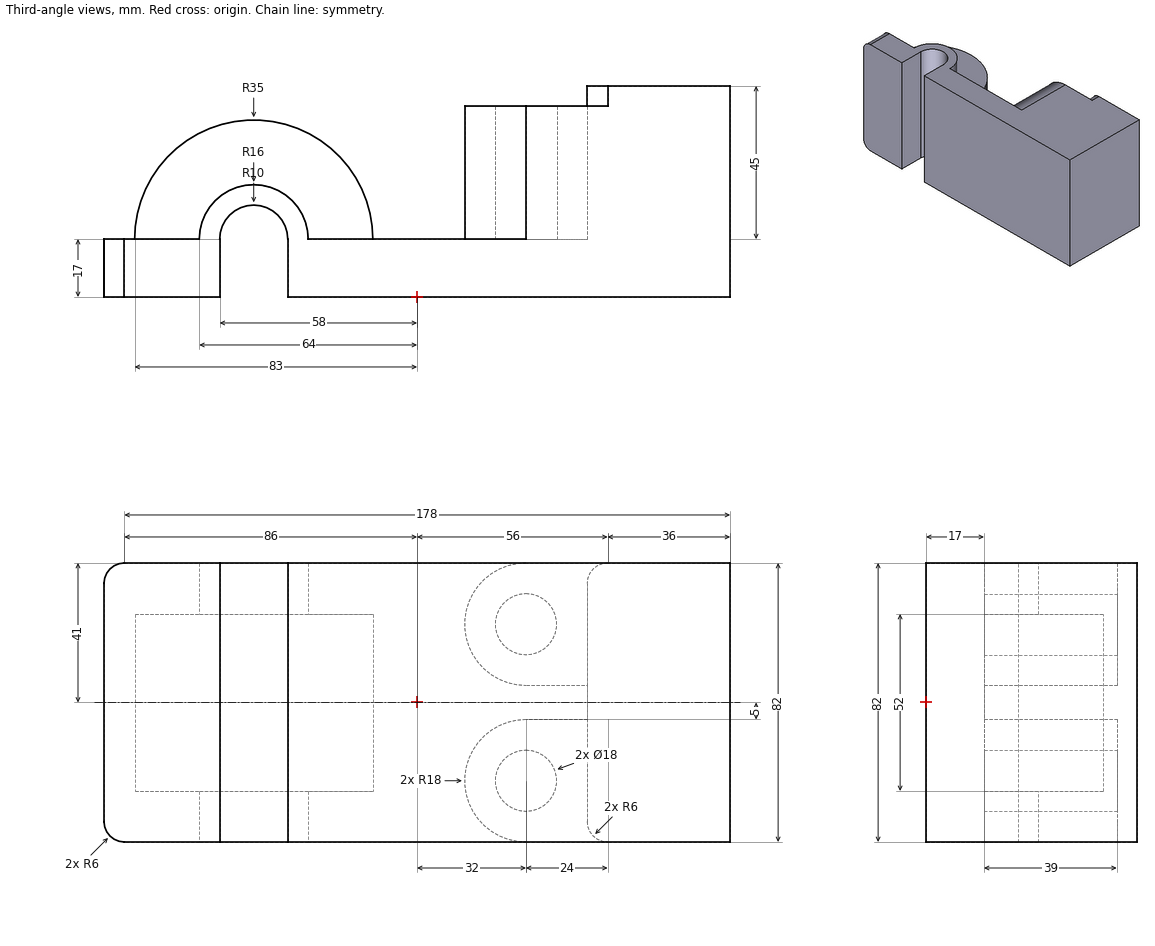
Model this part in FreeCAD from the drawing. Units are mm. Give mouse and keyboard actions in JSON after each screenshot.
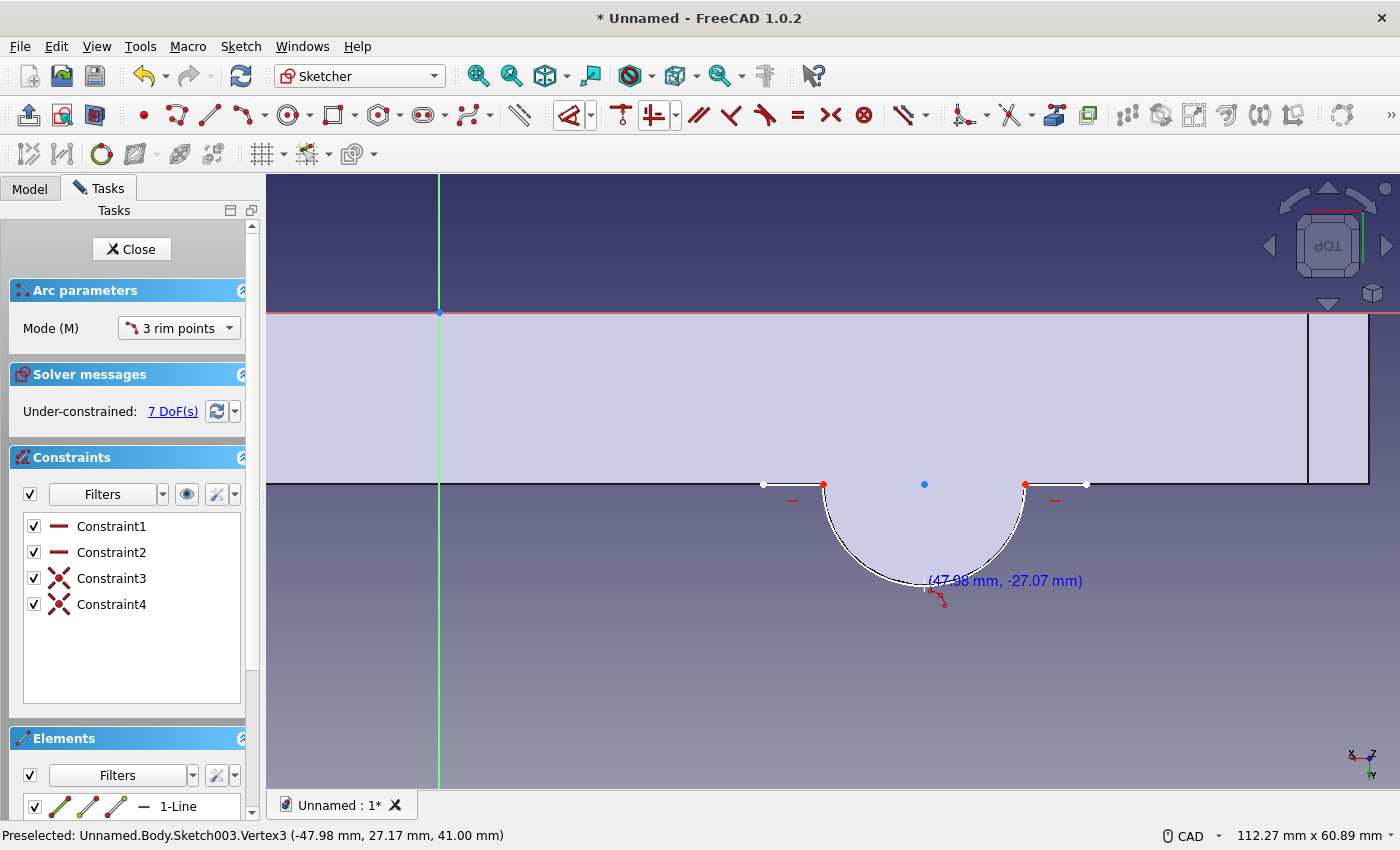
{"action": "left_click", "coordinate": [763, 485]}
{"action": "left_click", "coordinate": [1086, 485]}
{"action": "left_click", "coordinate": [924, 646]}
{"action": "key", "text": "Escape"}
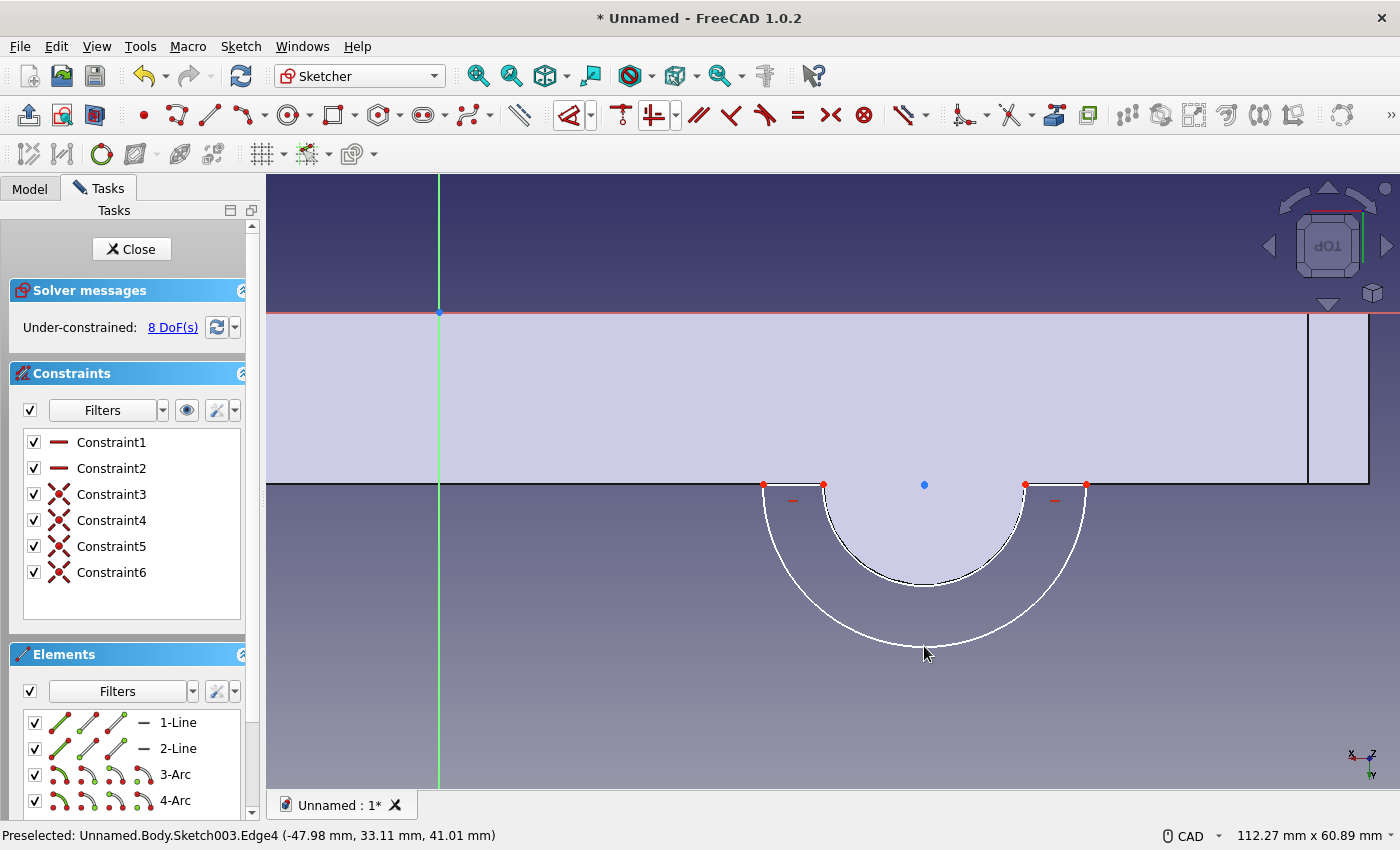
{"action": "left_click", "coordinate": [865, 567]}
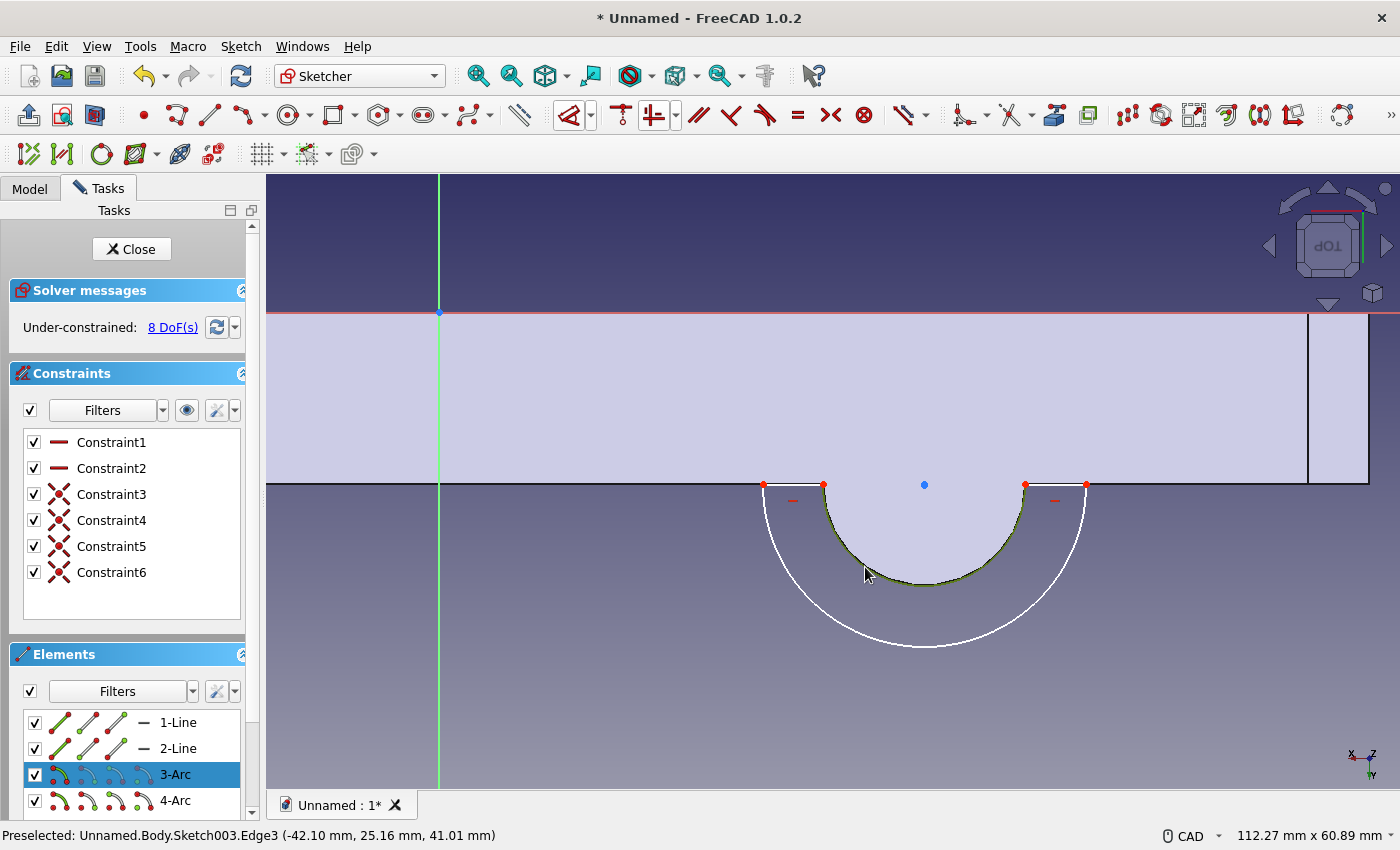
{"action": "left_click", "coordinate": [829, 616]}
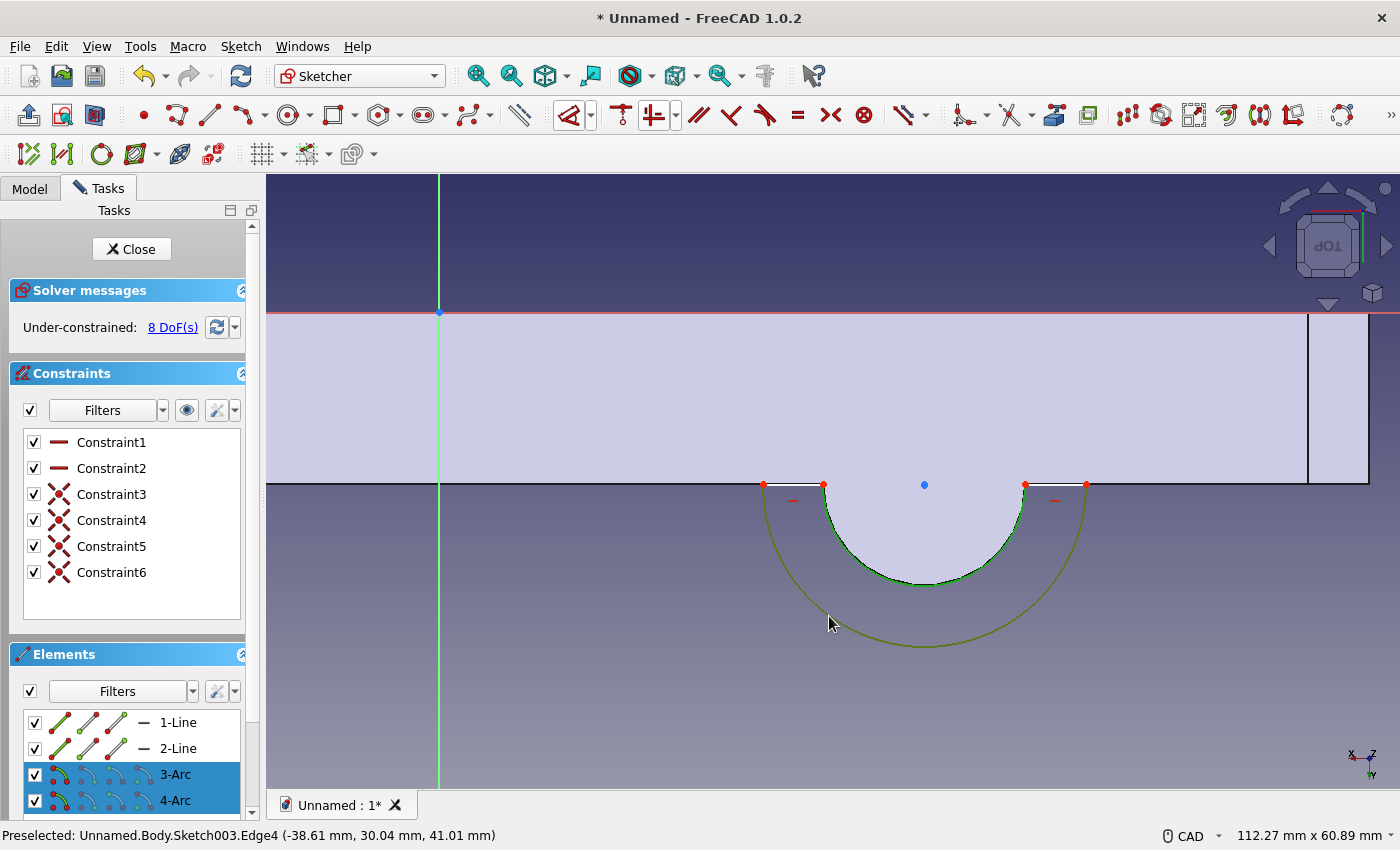
{"action": "left_click", "coordinate": [621, 116]}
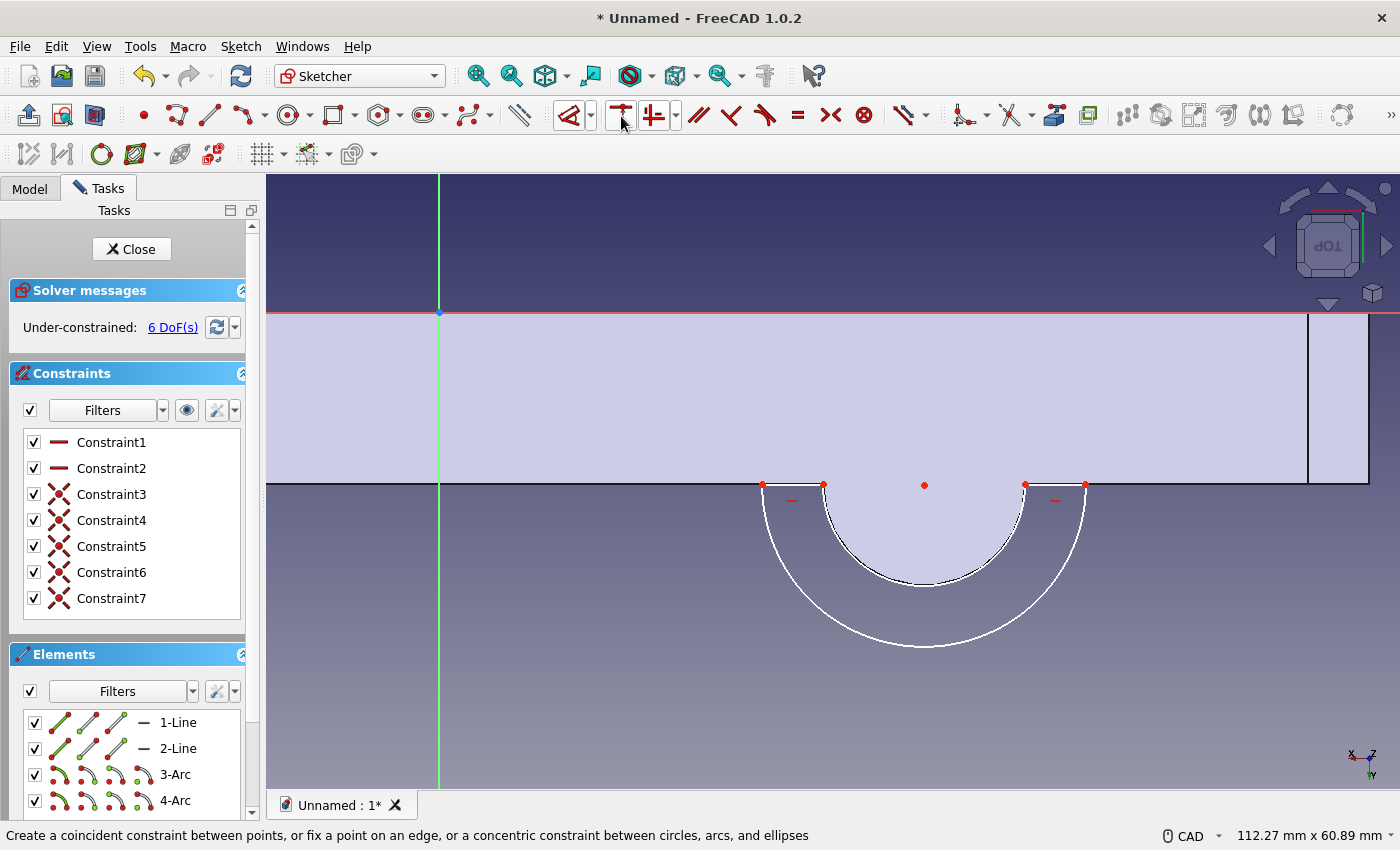
{"action": "left_click", "coordinate": [865, 567]}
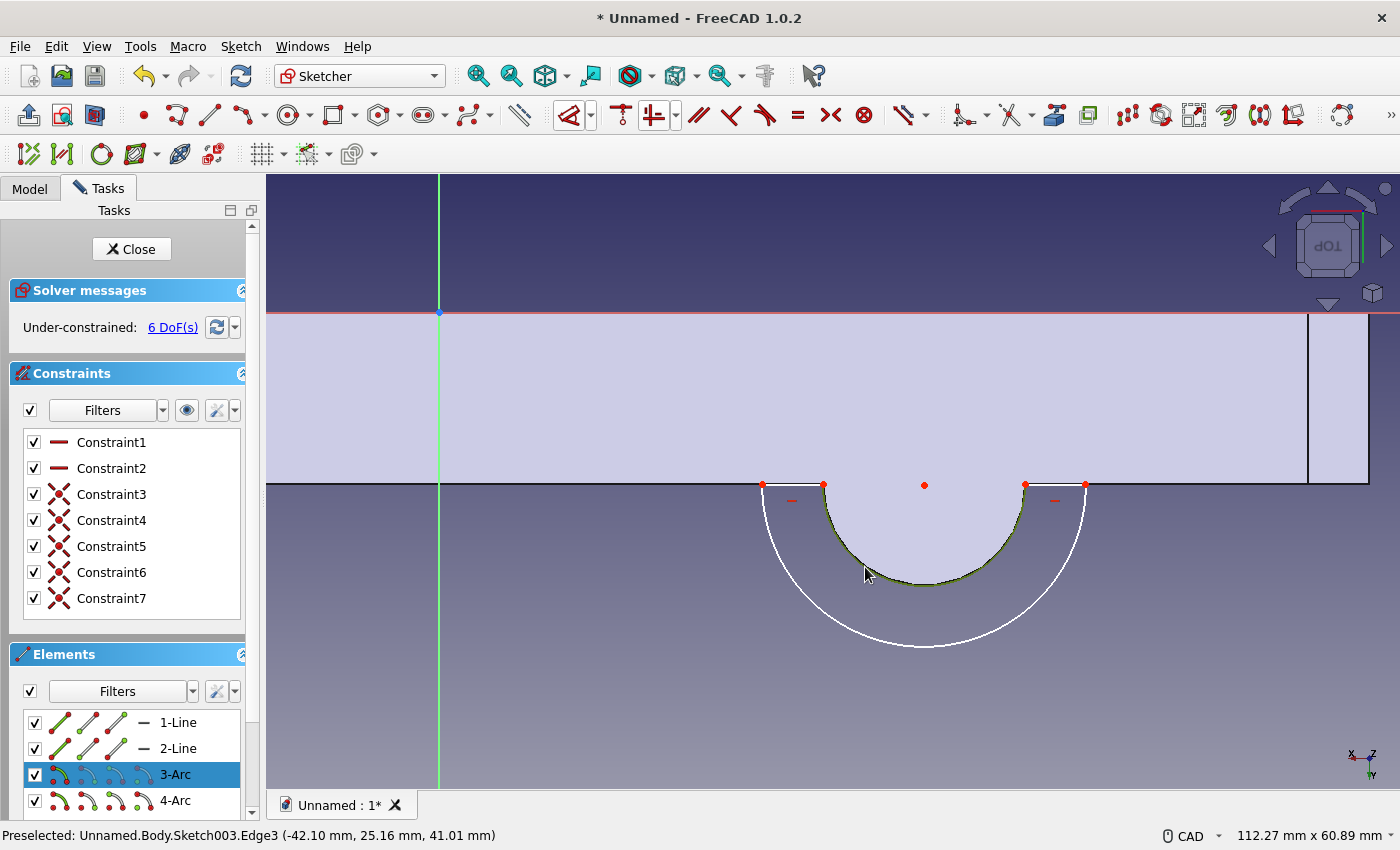
{"action": "left_click", "coordinate": [590, 116]}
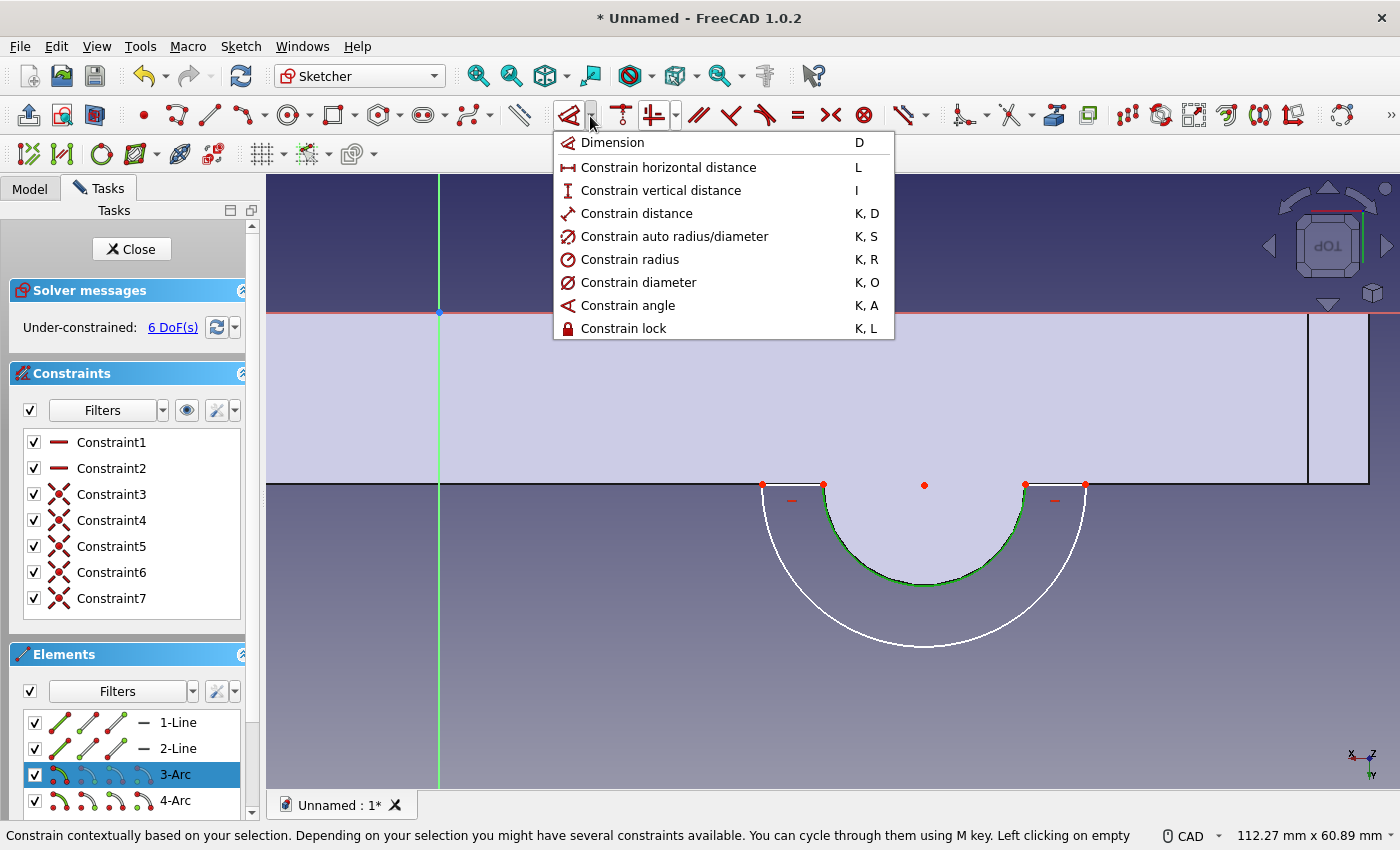
{"action": "left_click", "coordinate": [724, 260]}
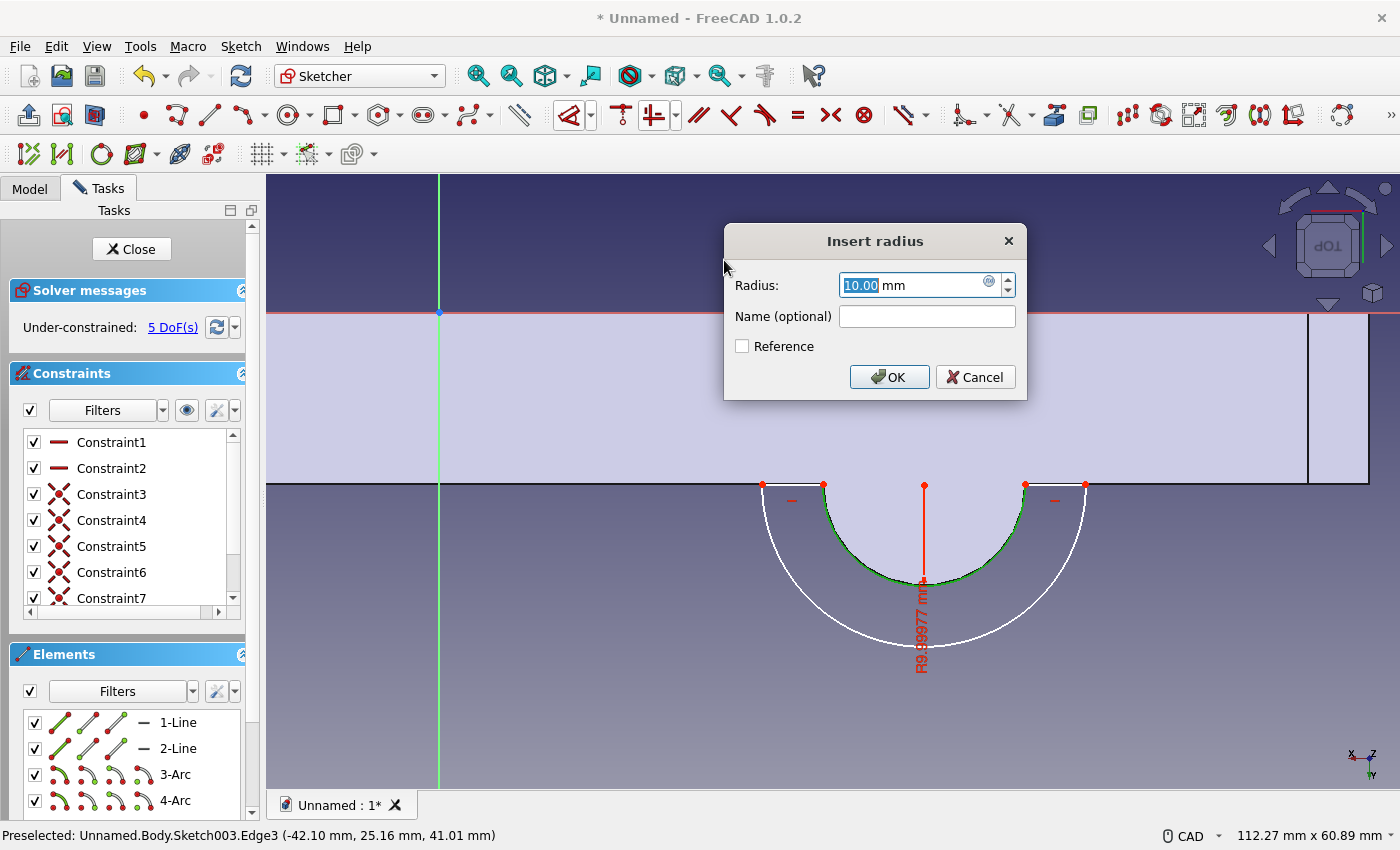
{"action": "type", "text": "10"}
{"action": "key", "text": "Return"}